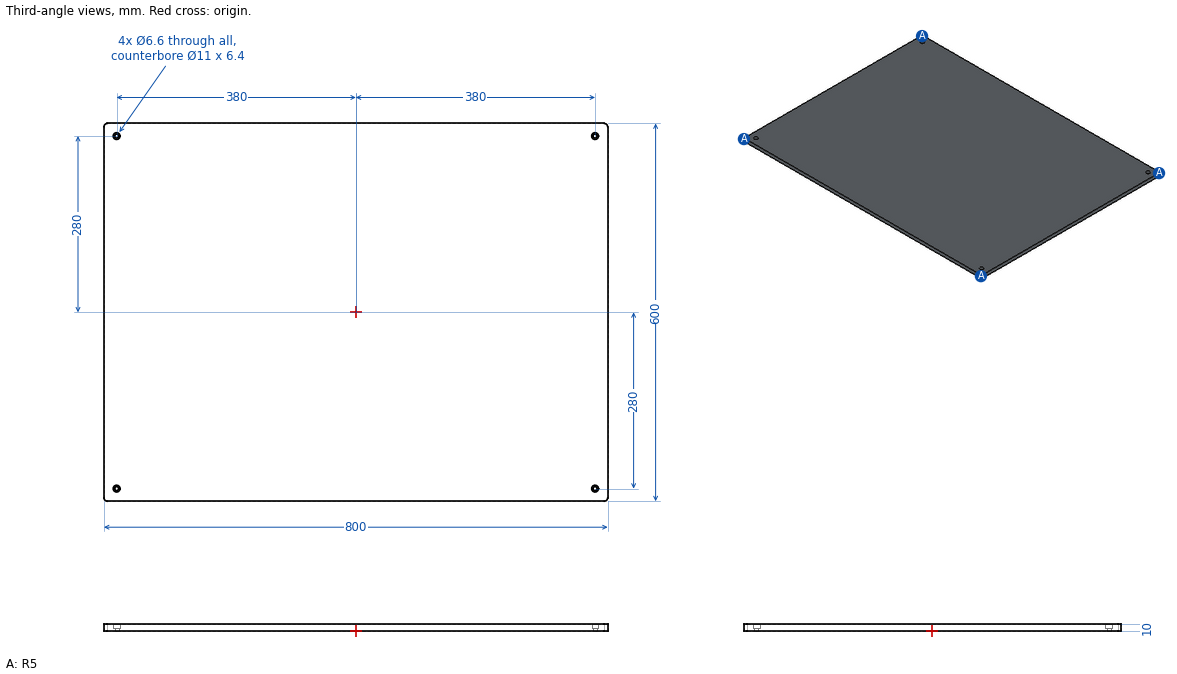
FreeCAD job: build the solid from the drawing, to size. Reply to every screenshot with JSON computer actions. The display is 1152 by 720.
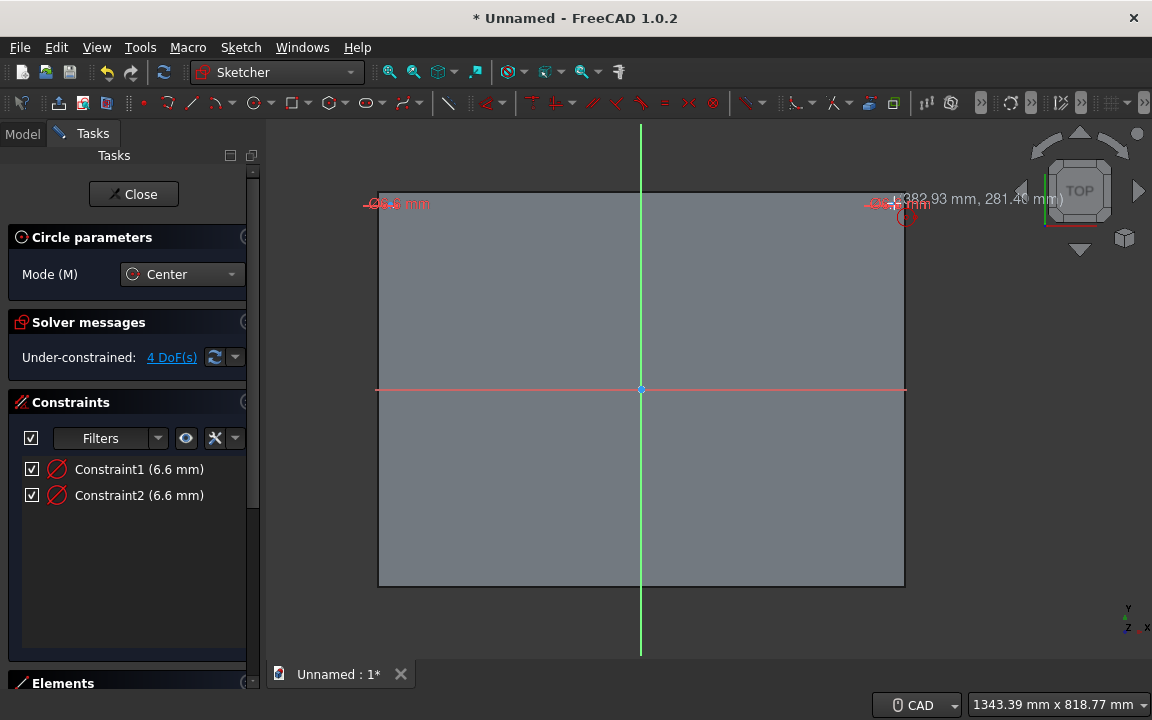
{"action": "scroll", "coordinate": [892, 574], "scroll_direction": "up", "scroll_amount": 12}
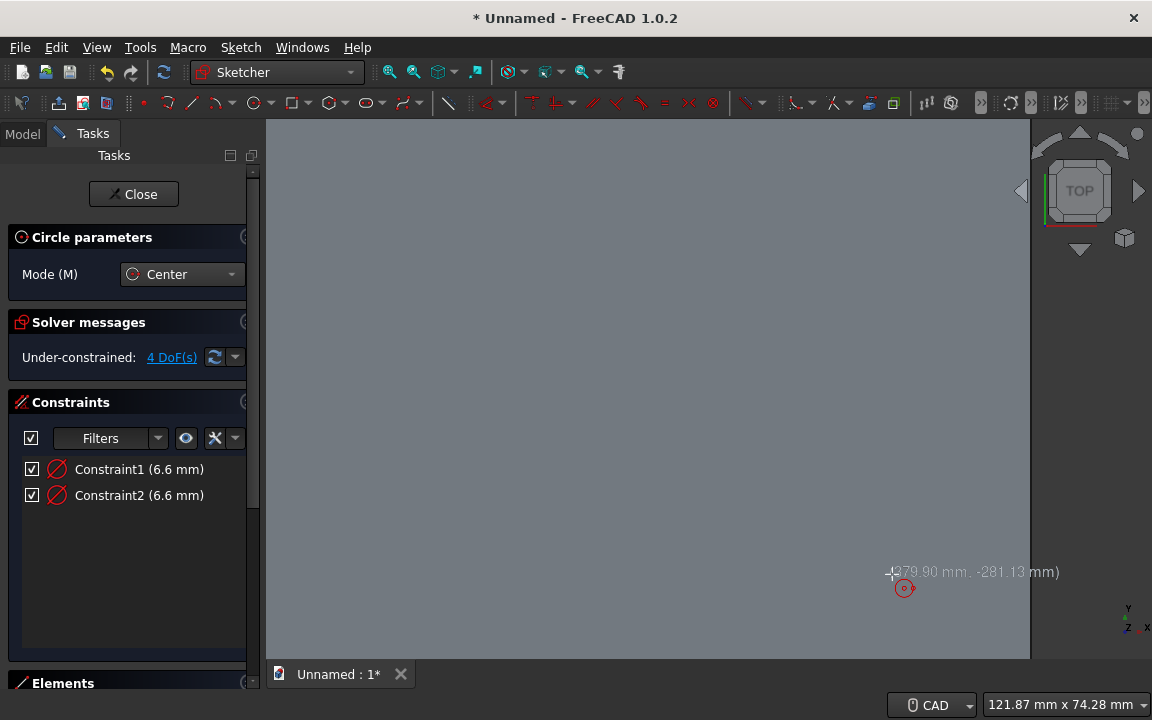
{"action": "scroll", "coordinate": [892, 574], "scroll_direction": "down", "scroll_amount": 12}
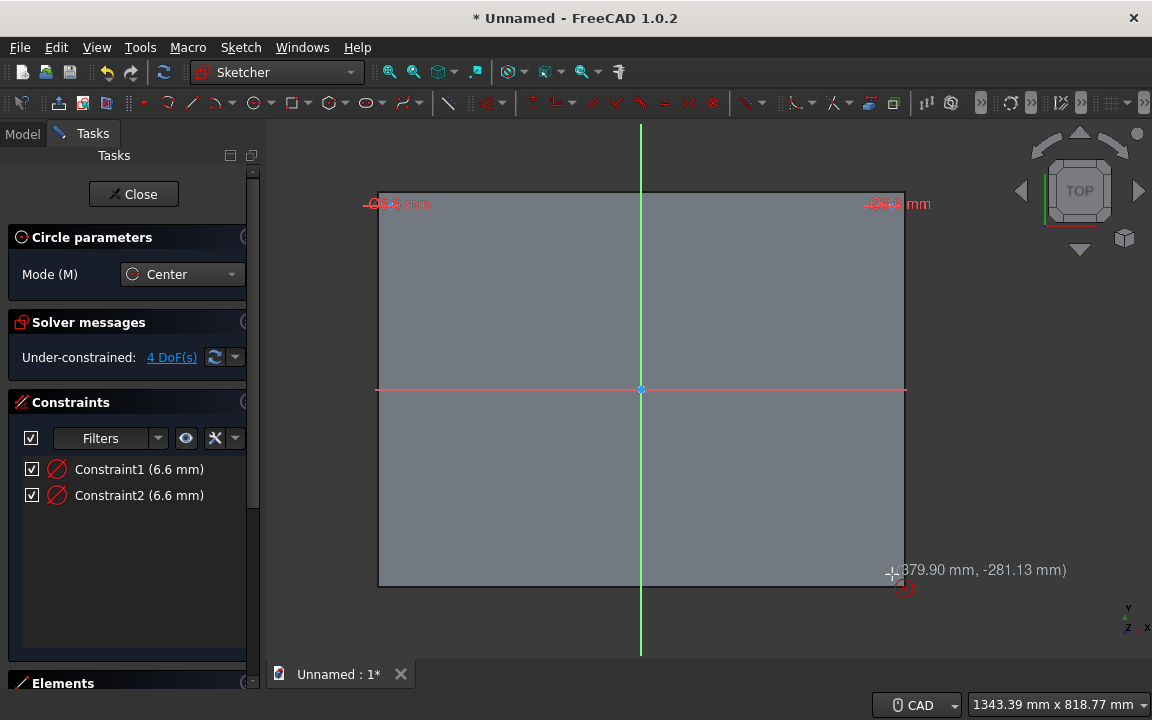
{"action": "left_click", "coordinate": [892, 574]}
{"action": "mouse_move", "coordinate": [894, 573]}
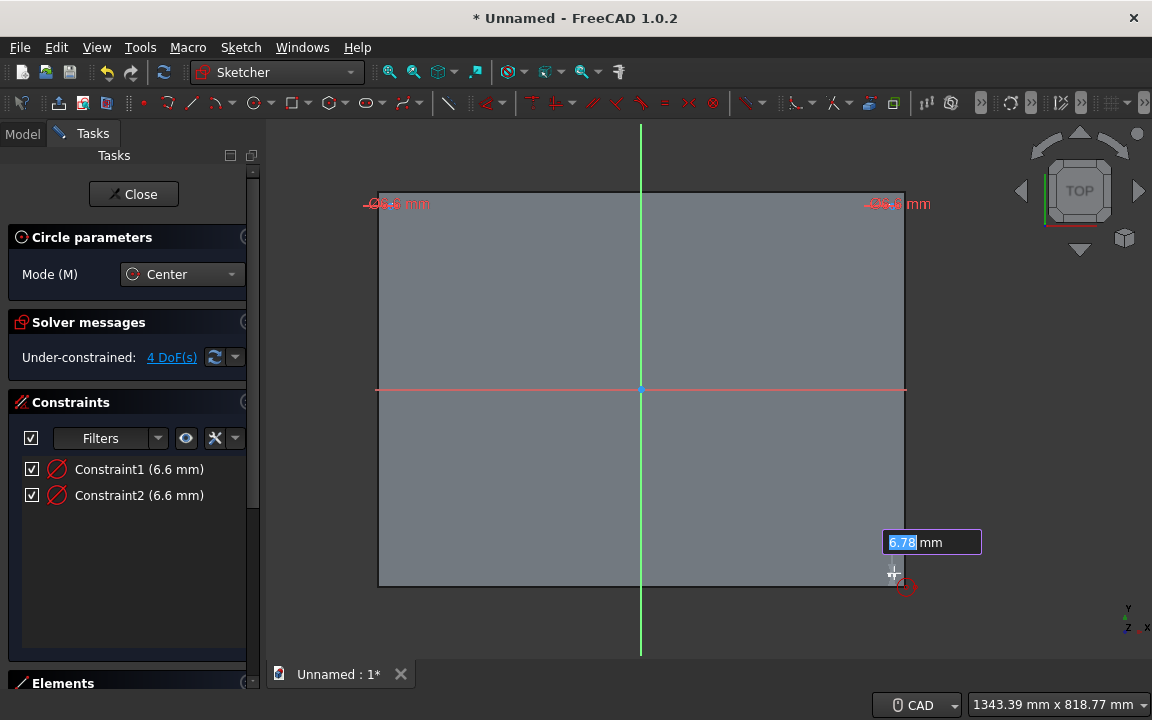
{"action": "type", "text": "6.6"}
{"action": "key", "text": "Return"}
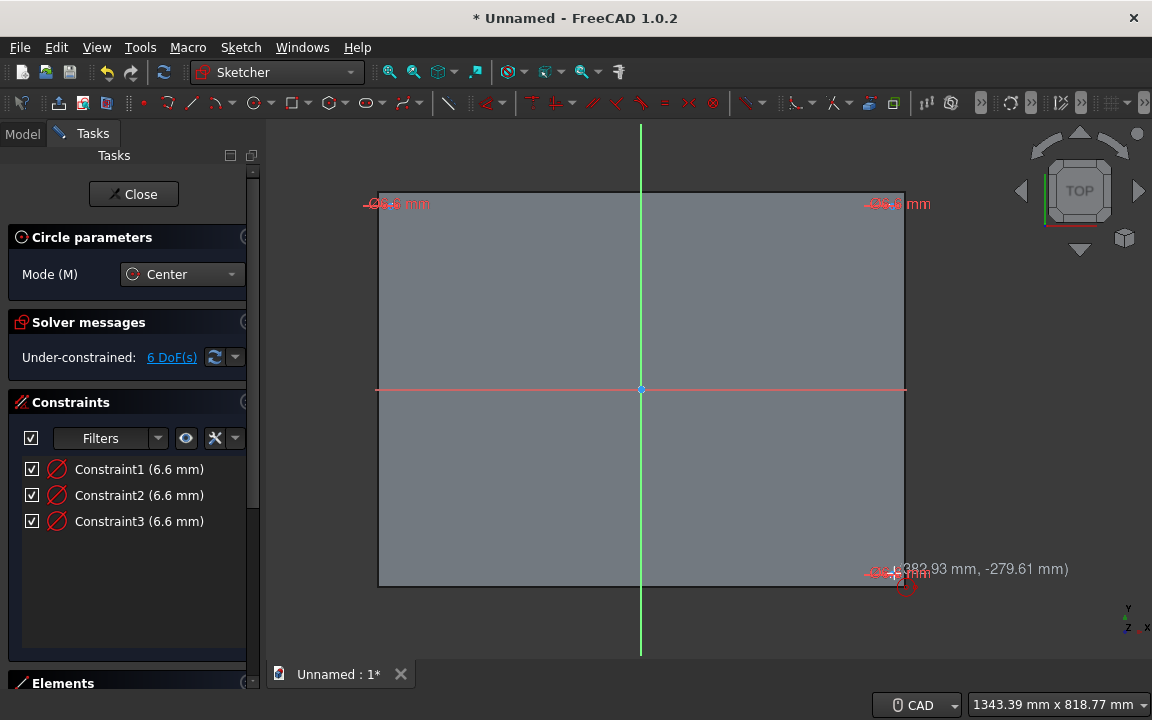
{"action": "scroll", "coordinate": [391, 574], "scroll_direction": "up", "scroll_amount": 12}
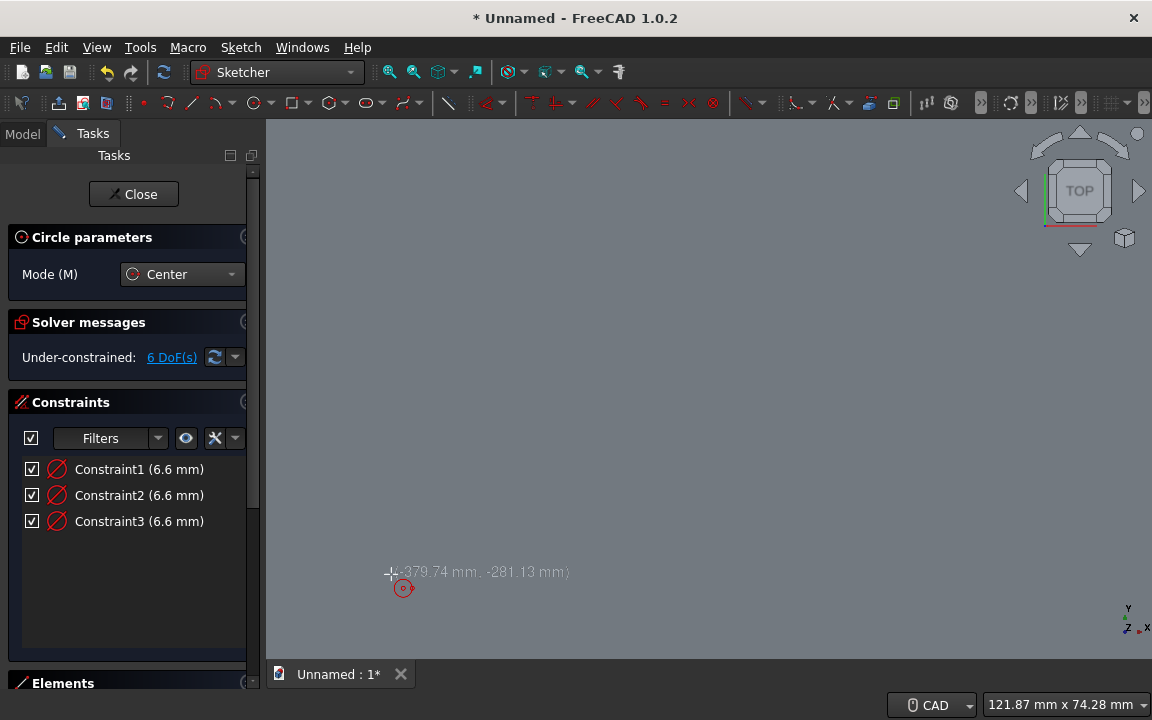
{"action": "scroll", "coordinate": [390, 574], "scroll_direction": "down", "scroll_amount": 12}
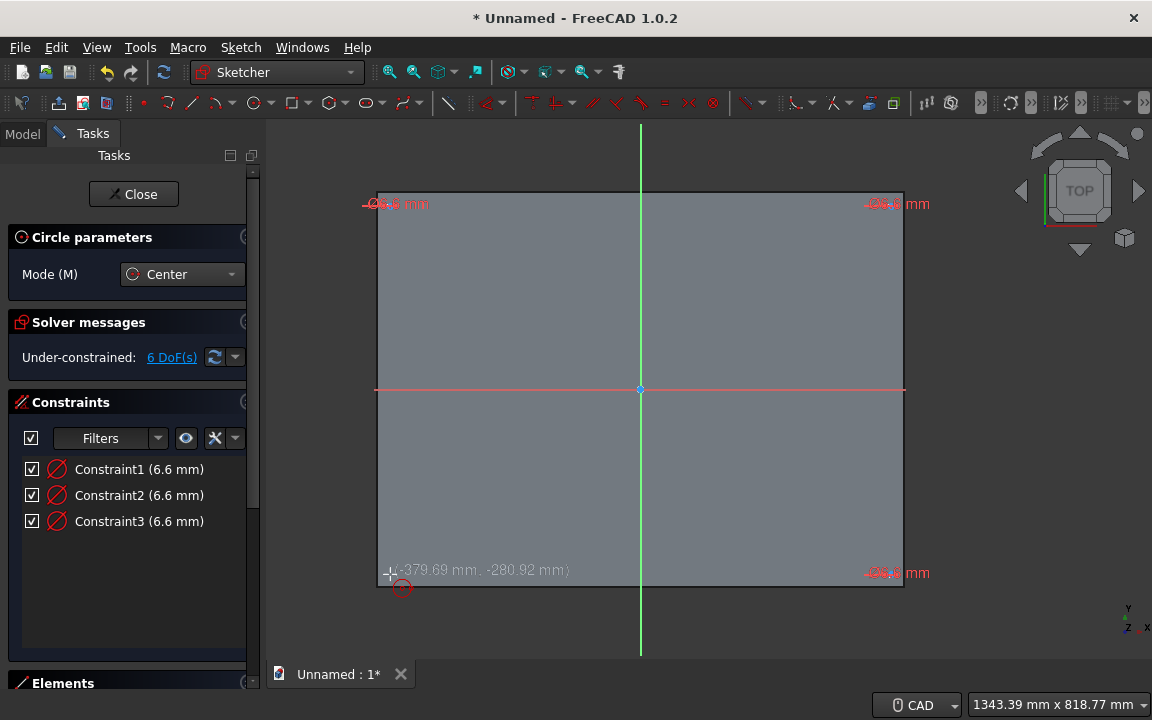
{"action": "left_click", "coordinate": [390, 574]}
{"action": "mouse_move", "coordinate": [391, 573]}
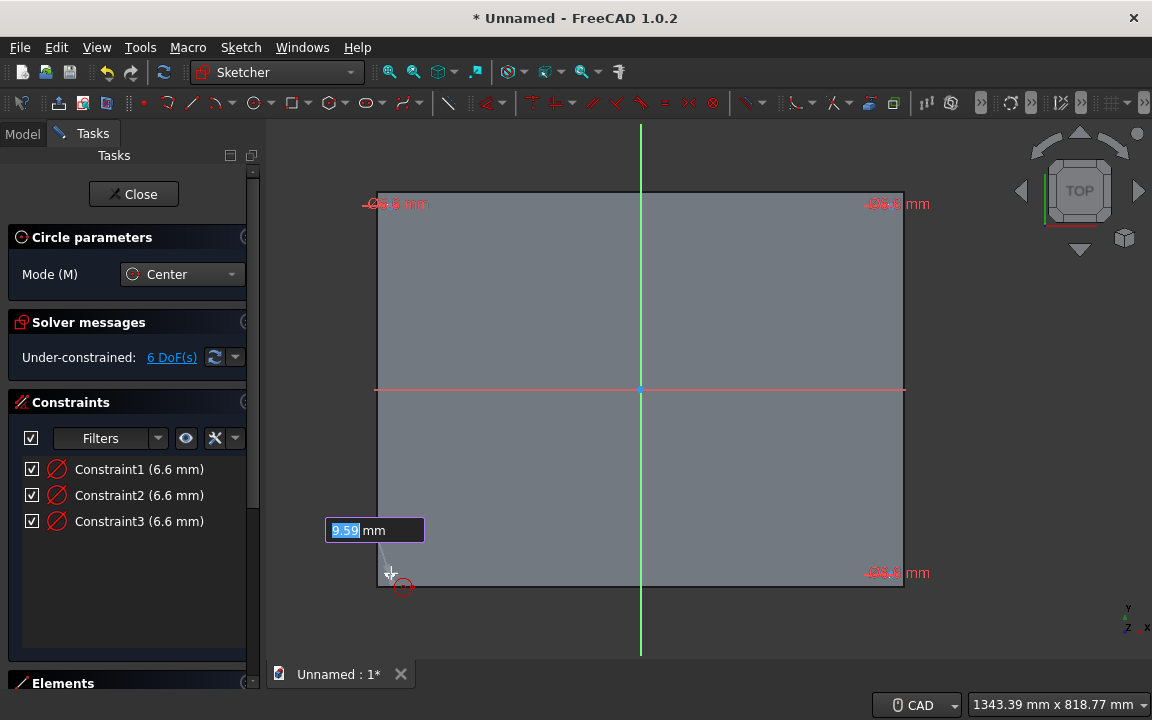
{"action": "type", "text": "6.6"}
{"action": "key", "text": "Return"}
{"action": "key", "text": "Escape"}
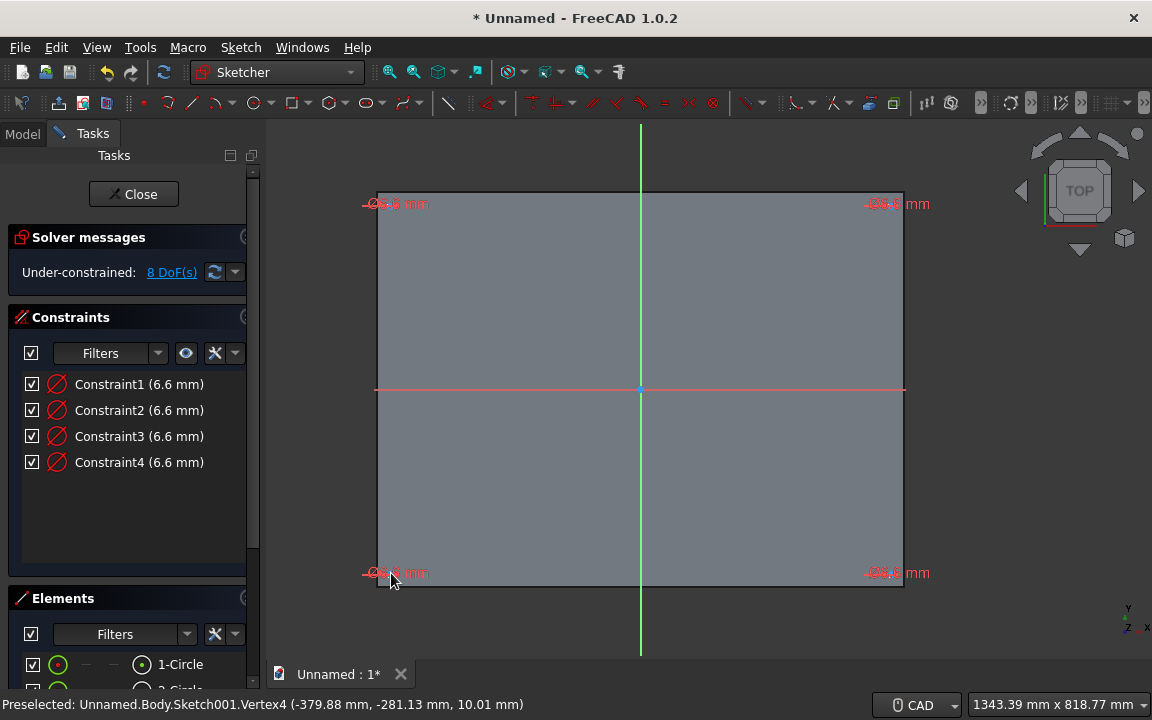
{"action": "left_click", "coordinate": [486, 104]}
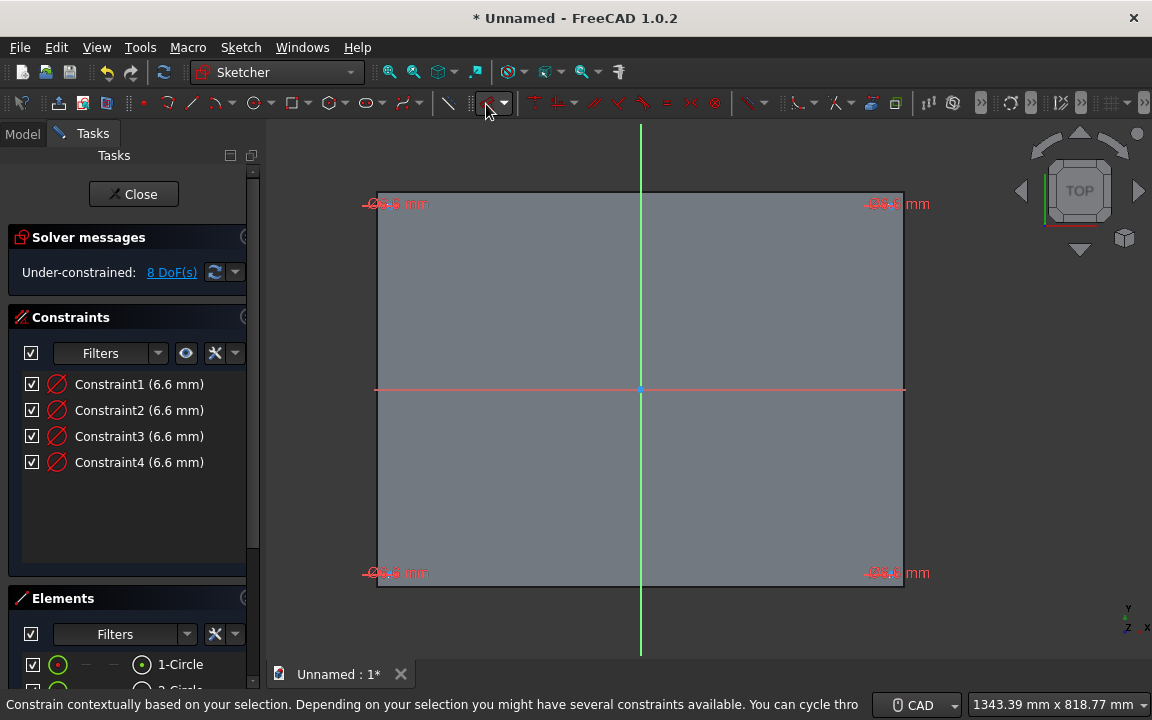
{"action": "left_click", "coordinate": [390, 206]}
{"action": "left_click", "coordinate": [515, 172]}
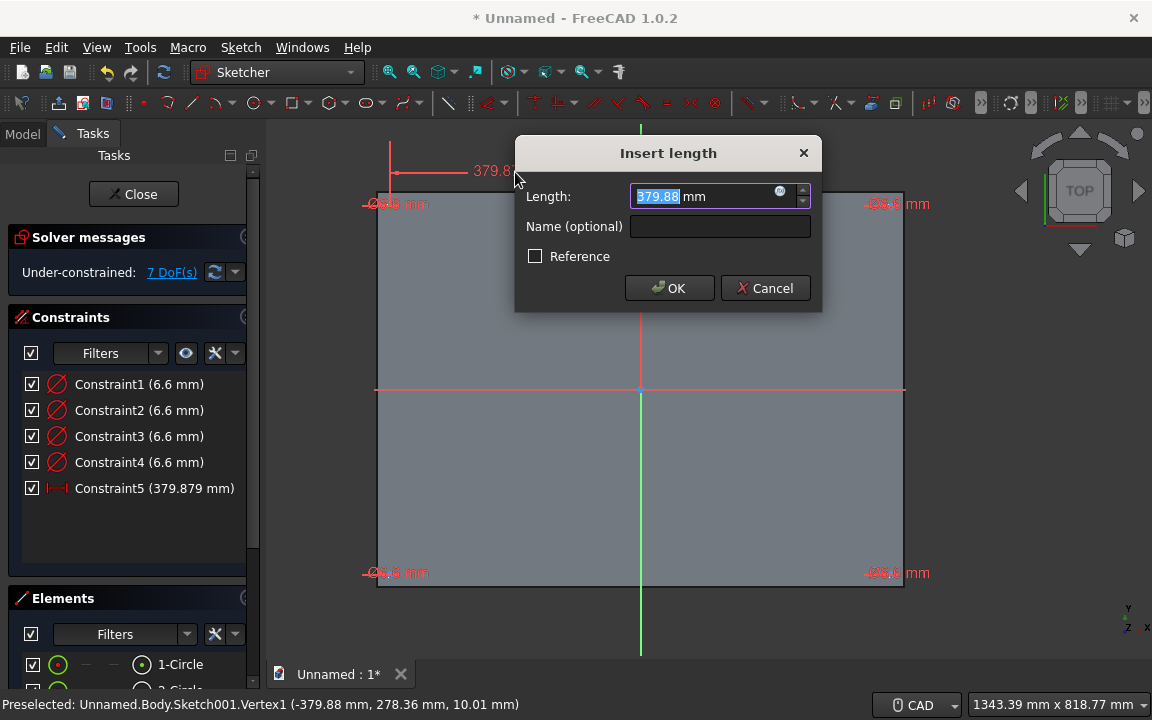
{"action": "type", "text": "380"}
{"action": "key", "text": "Return"}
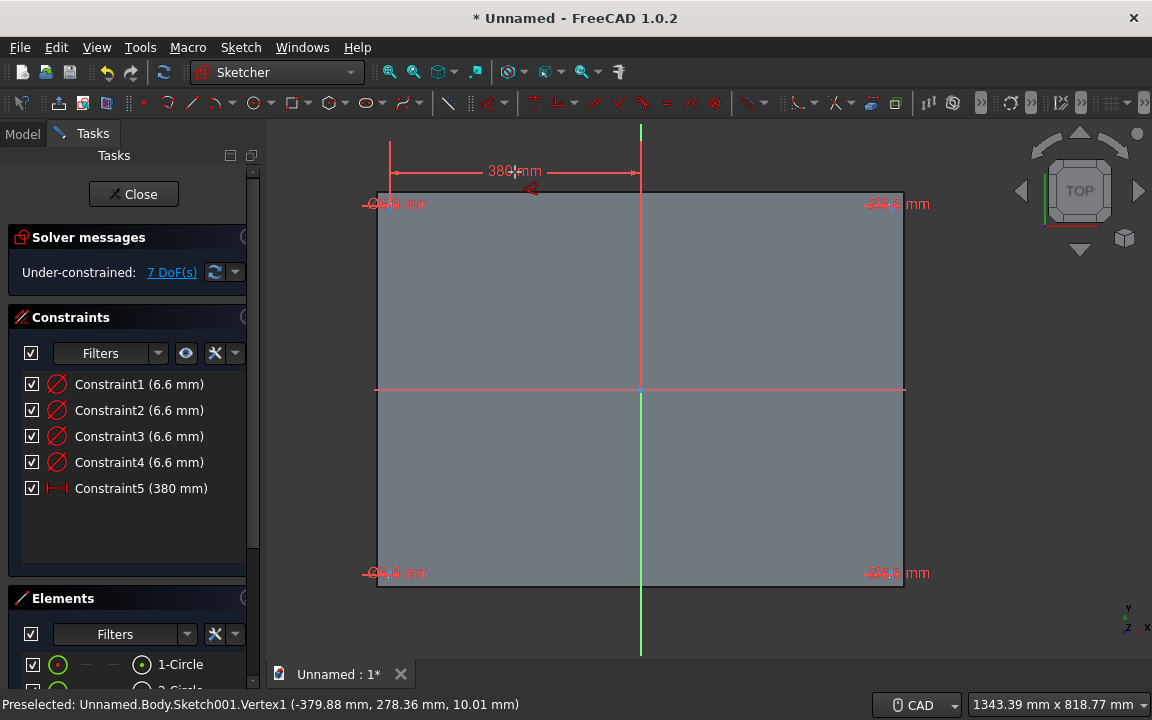
{"action": "left_click", "coordinate": [390, 206]}
{"action": "left_click", "coordinate": [356, 298]}